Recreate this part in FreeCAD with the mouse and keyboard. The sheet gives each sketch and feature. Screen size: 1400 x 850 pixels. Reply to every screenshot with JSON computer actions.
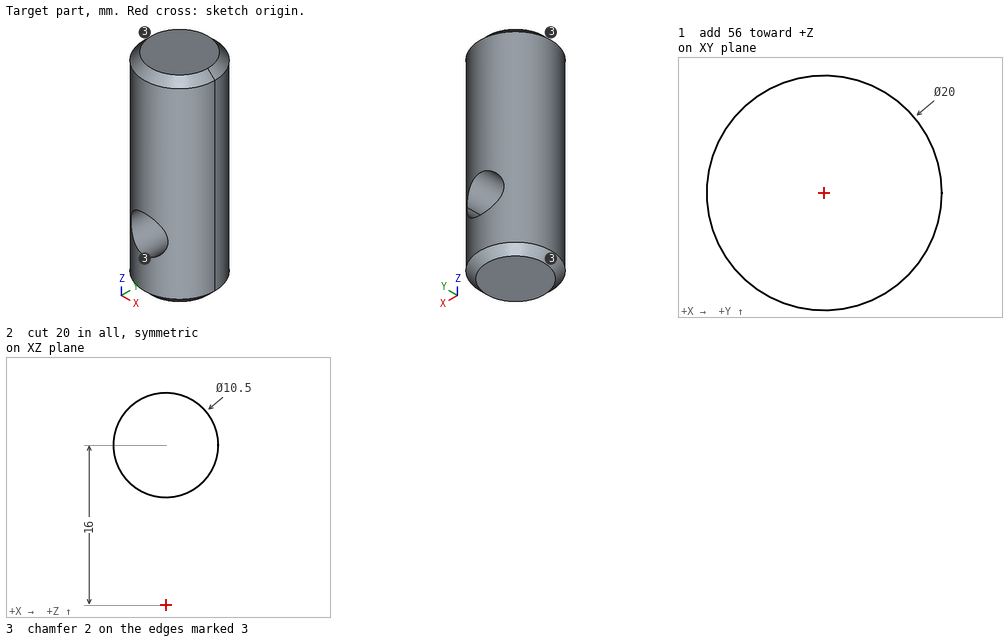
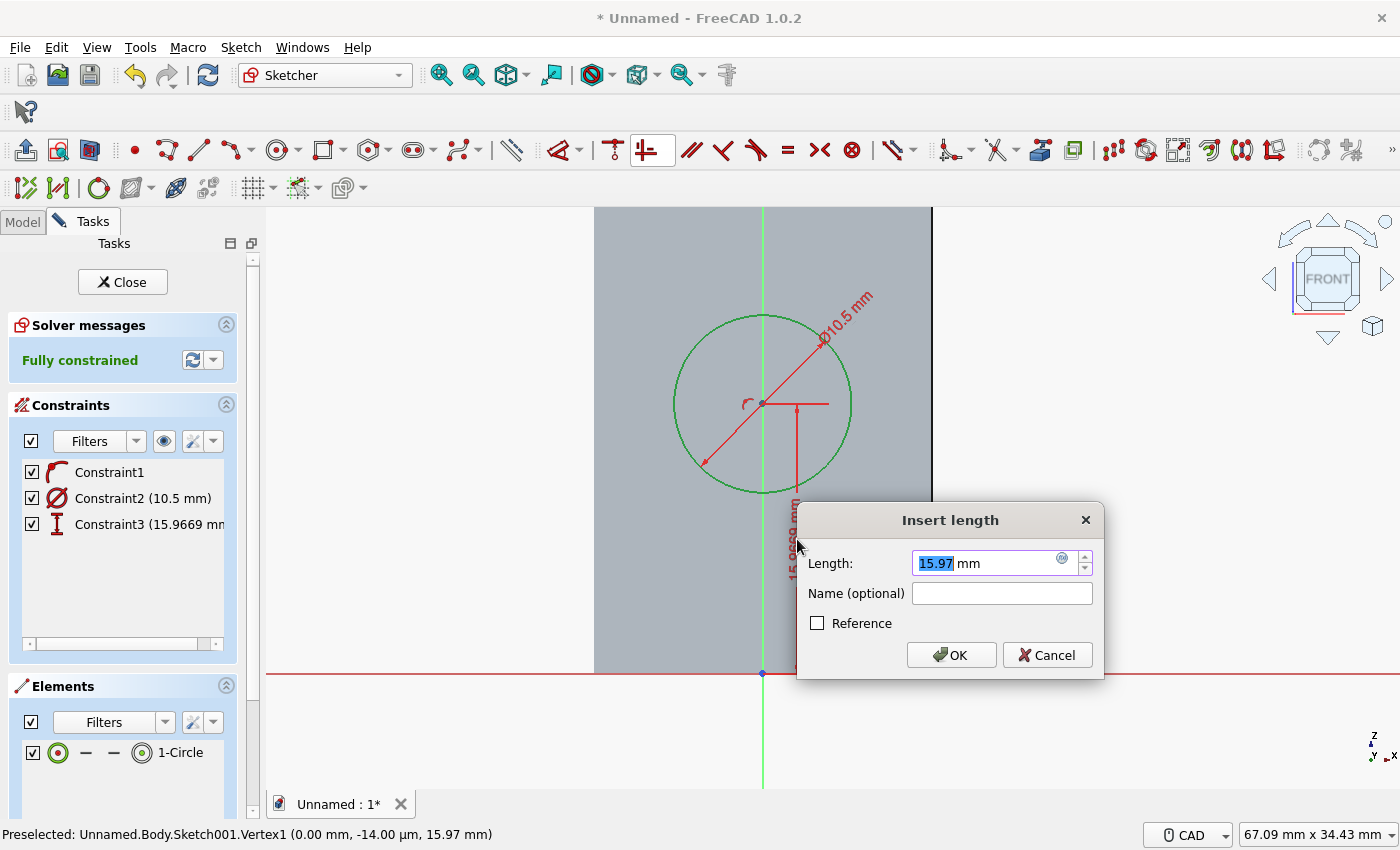
{"action": "type", "text": "16"}
{"action": "key", "text": "Return"}
{"action": "key", "text": "Escape"}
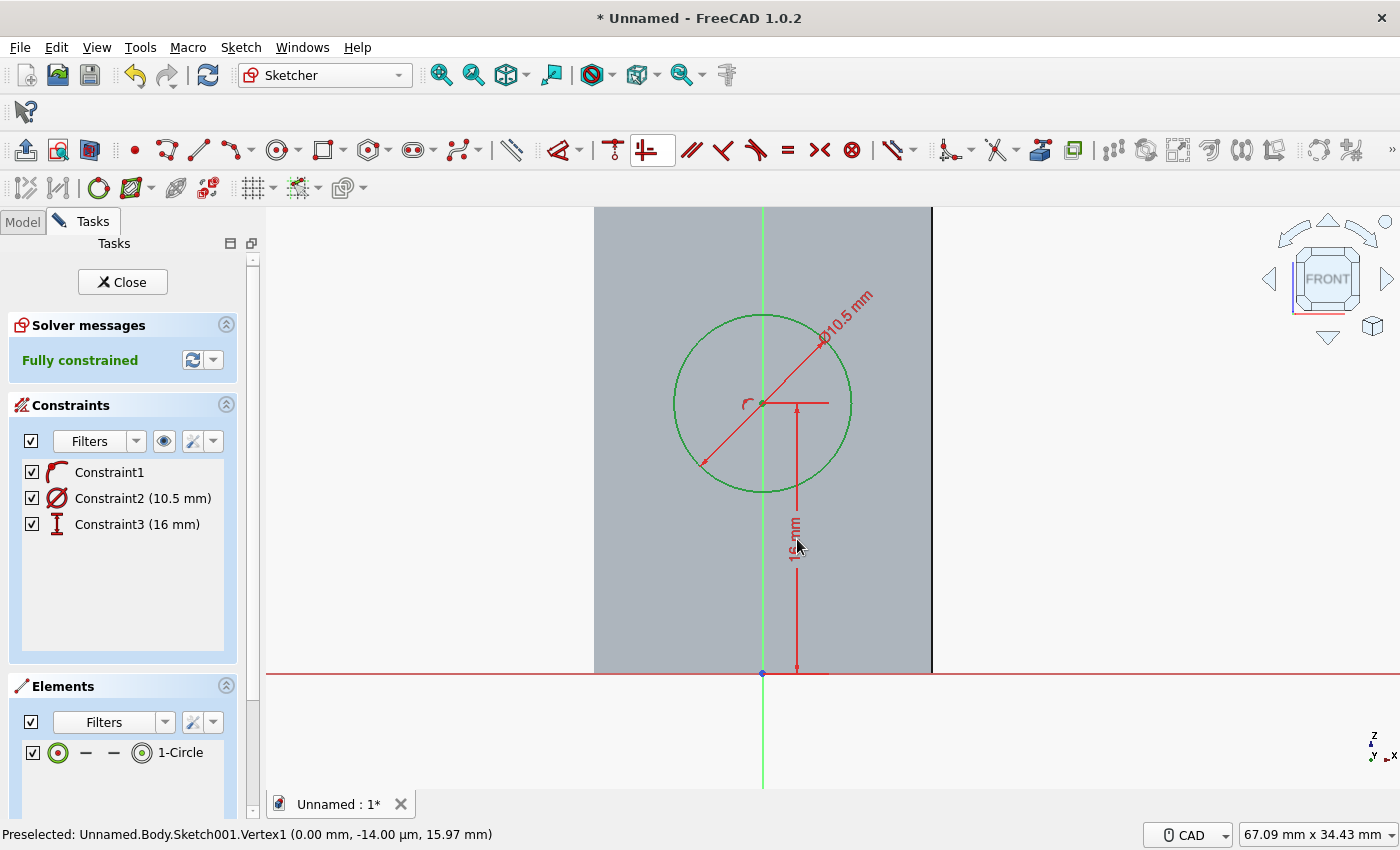
{"action": "left_click", "coordinate": [123, 282]}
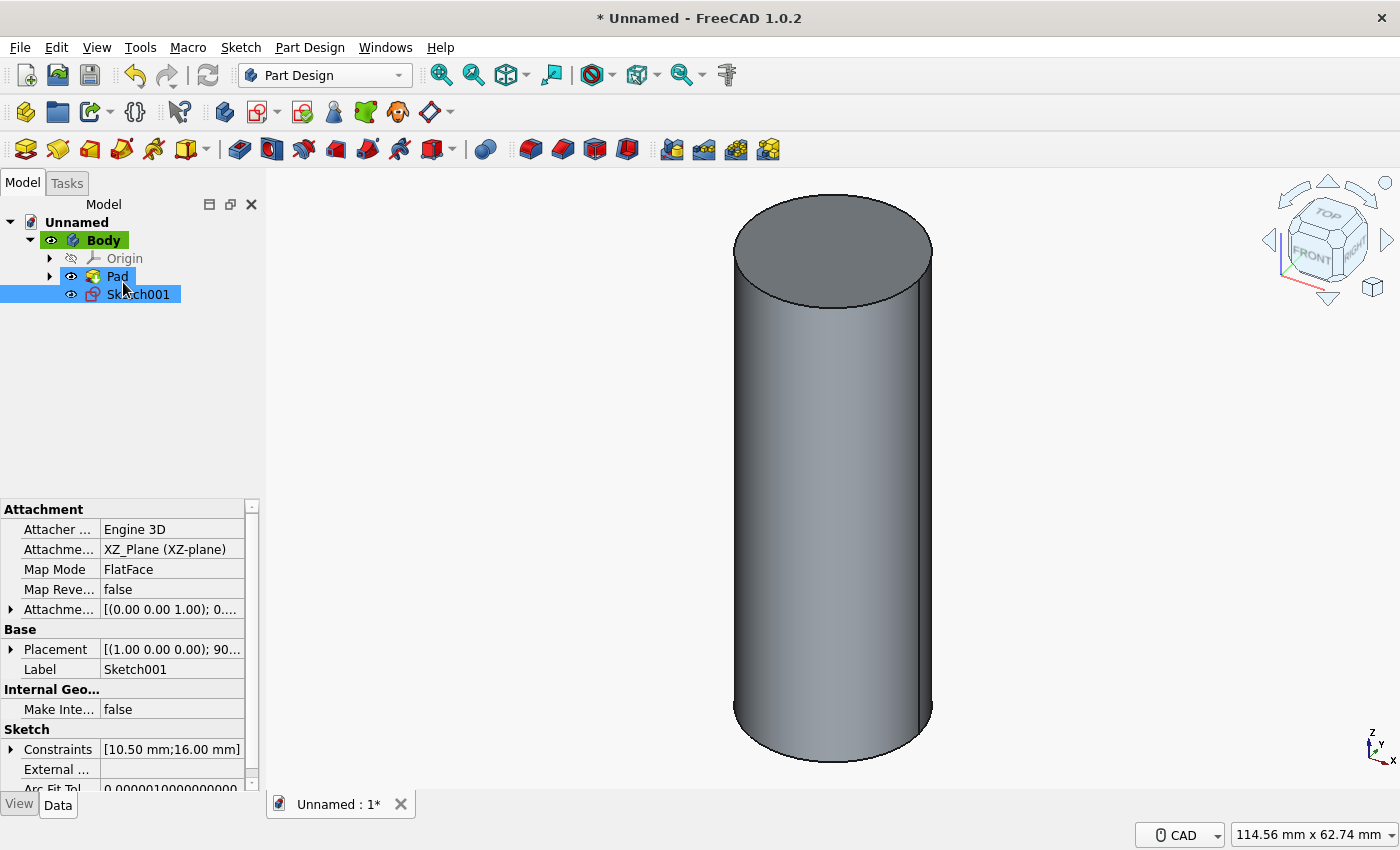
{"action": "left_click", "coordinate": [240, 150]}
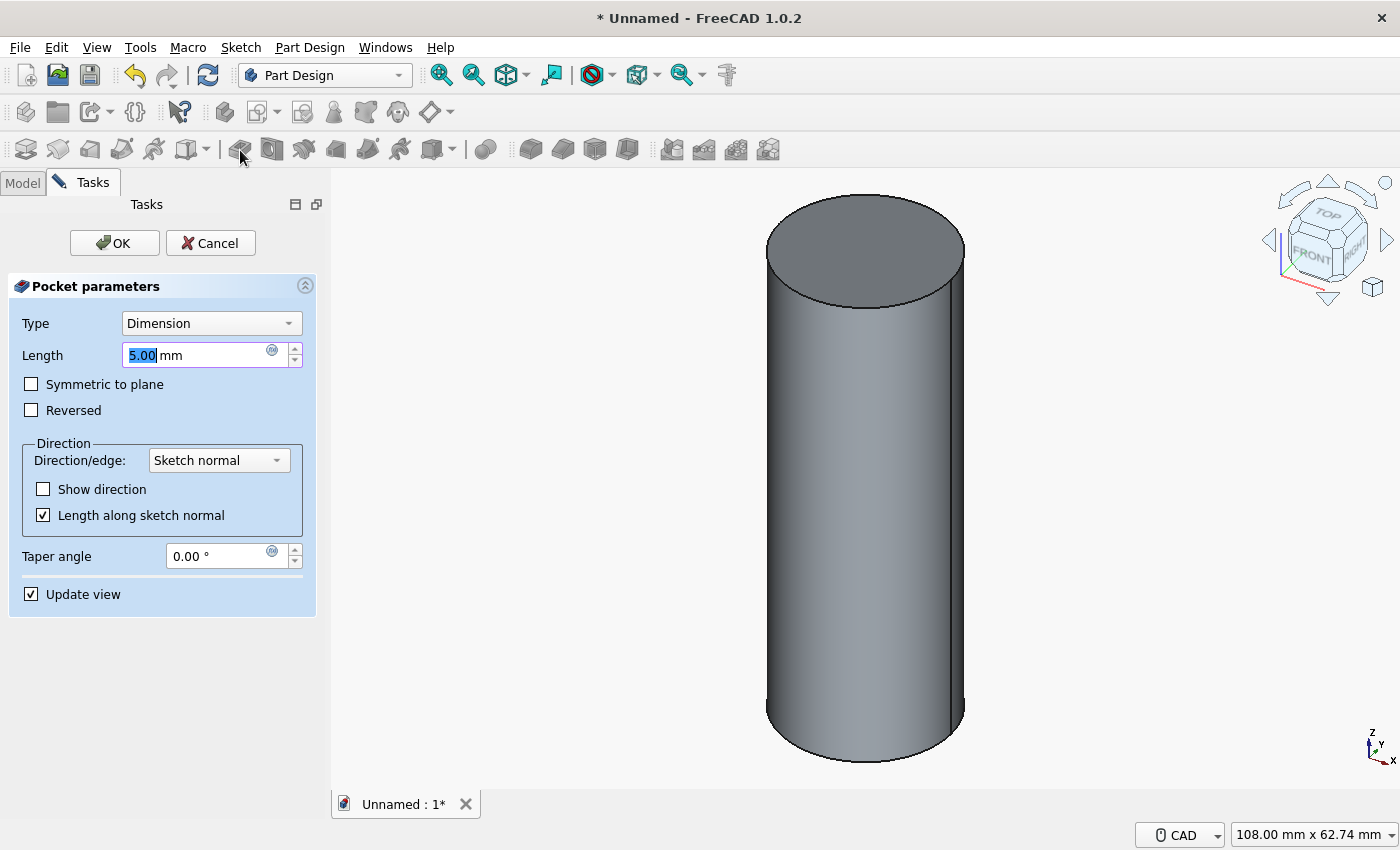
{"action": "type", "text": "20"}
{"action": "key", "text": "Tab"}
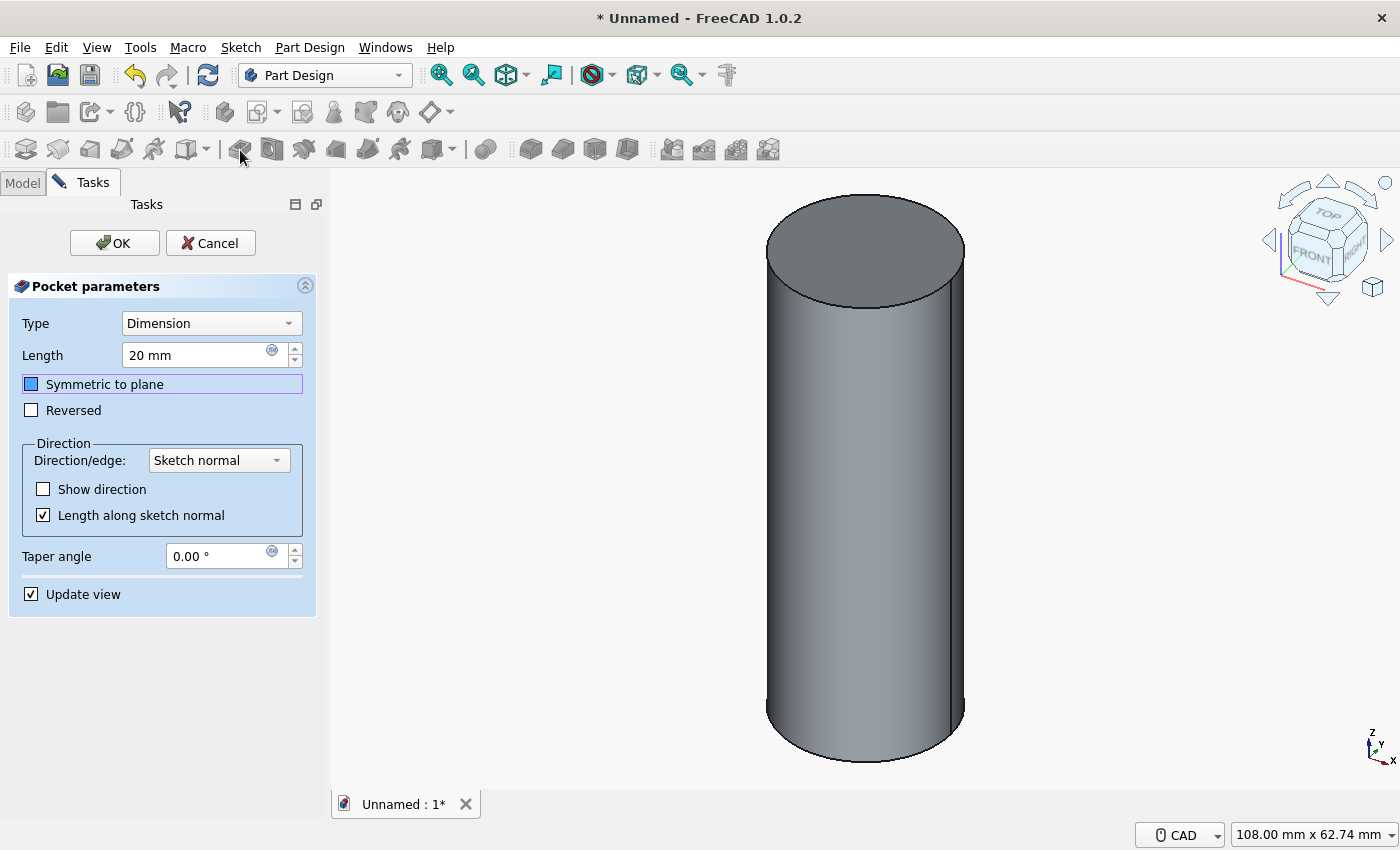
{"action": "left_click", "coordinate": [30, 384]}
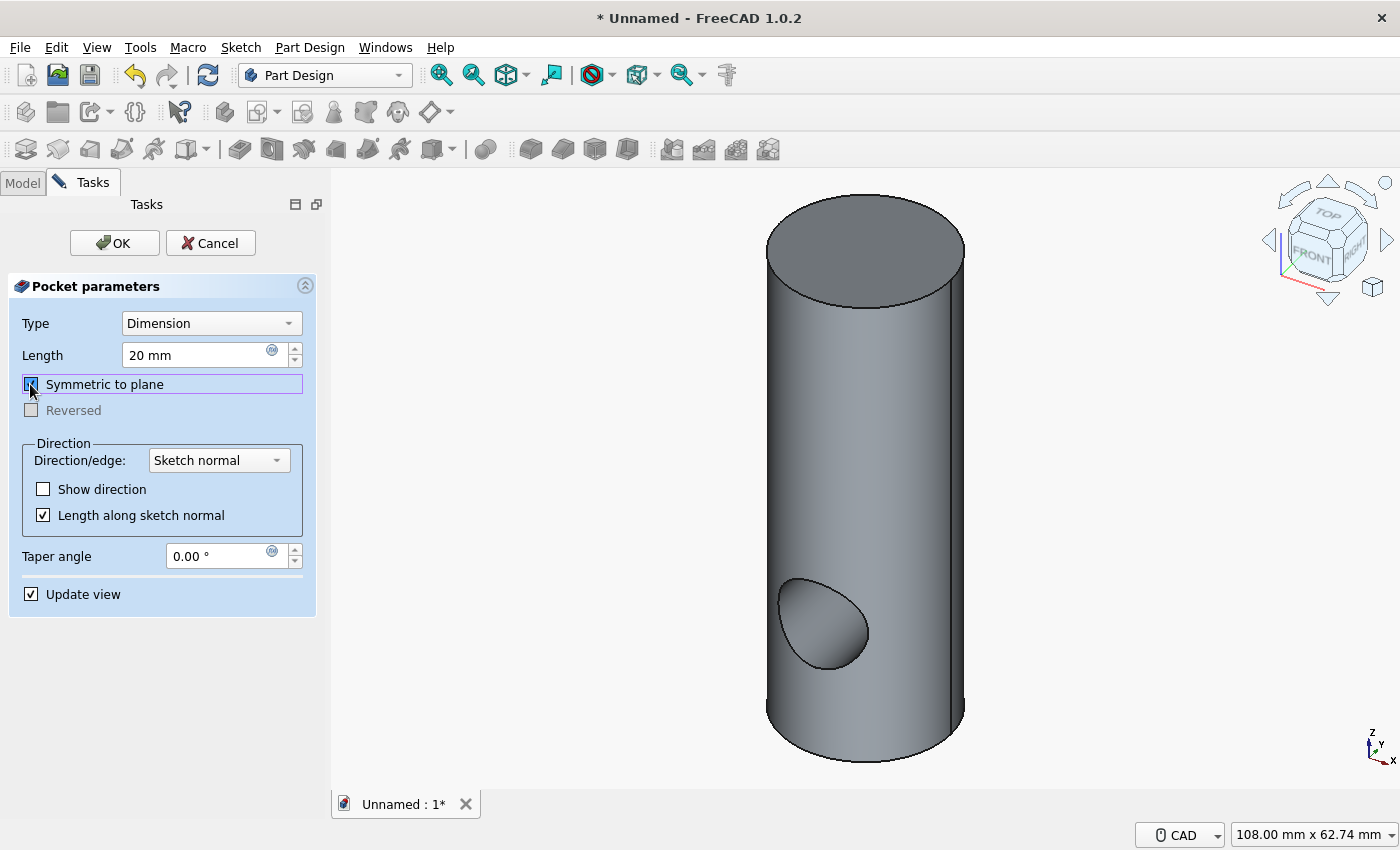
{"action": "left_click", "coordinate": [115, 243]}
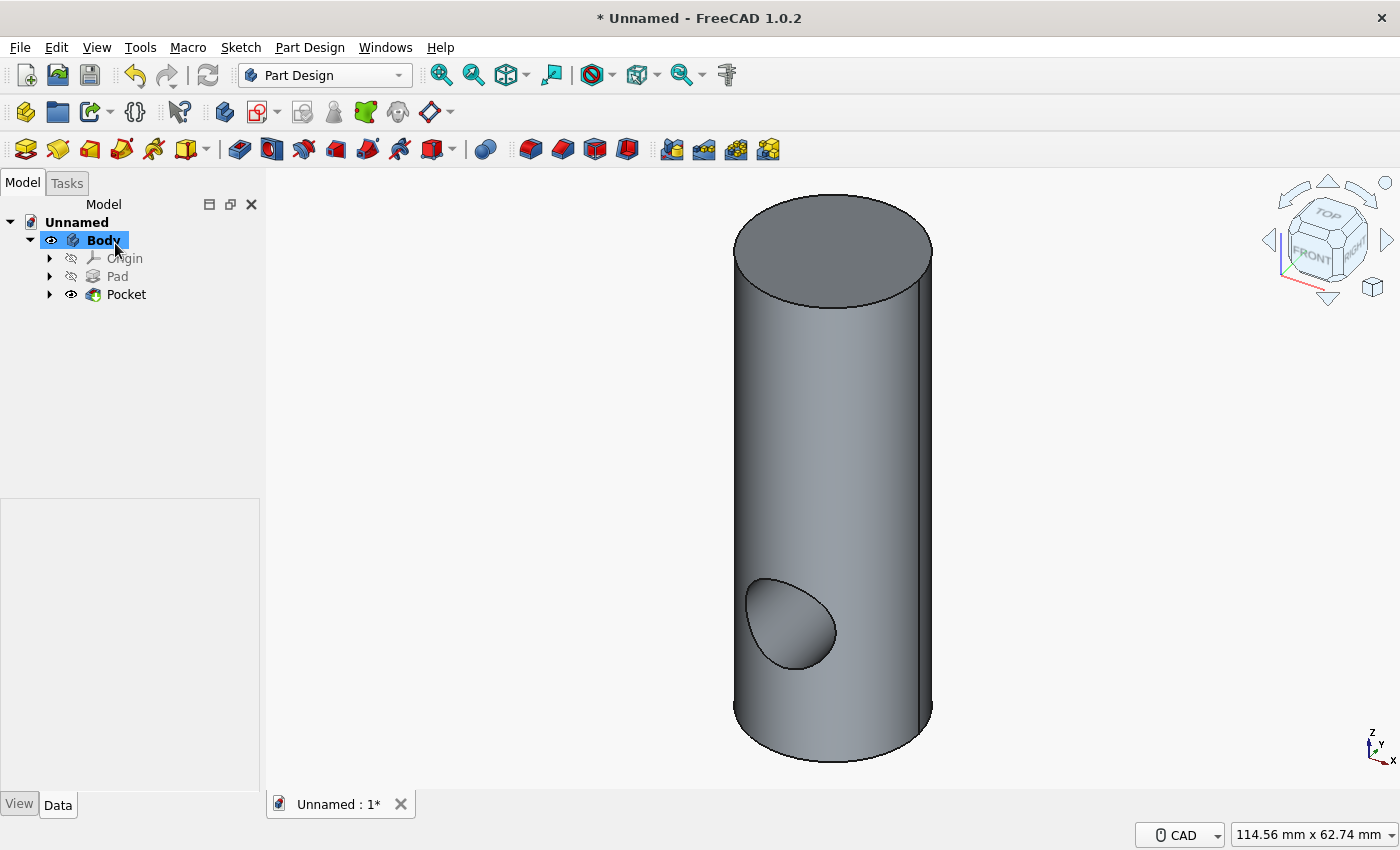
{"action": "left_click", "coordinate": [862, 759]}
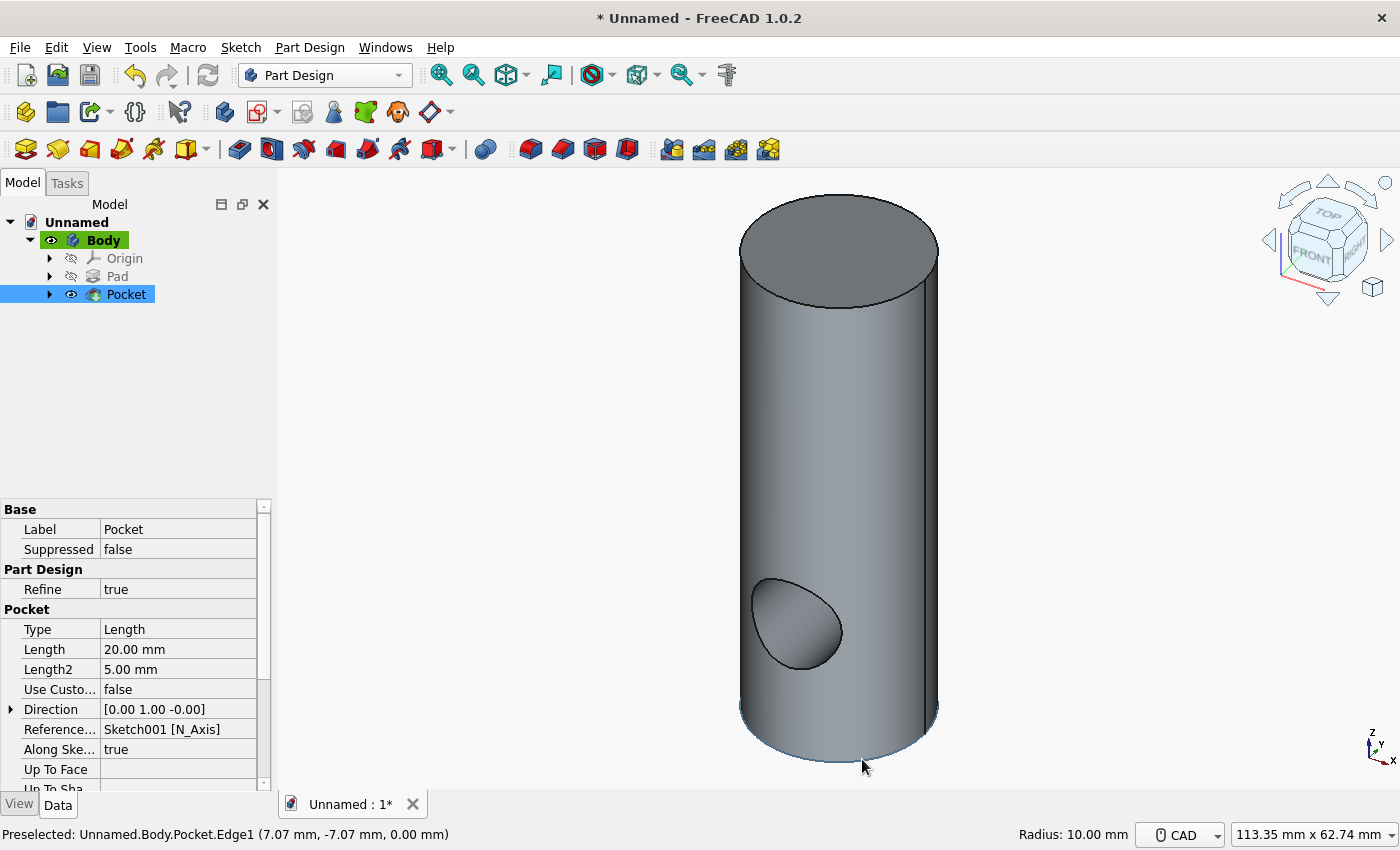
{"action": "left_click", "coordinate": [741, 256], "text": "ctrl"}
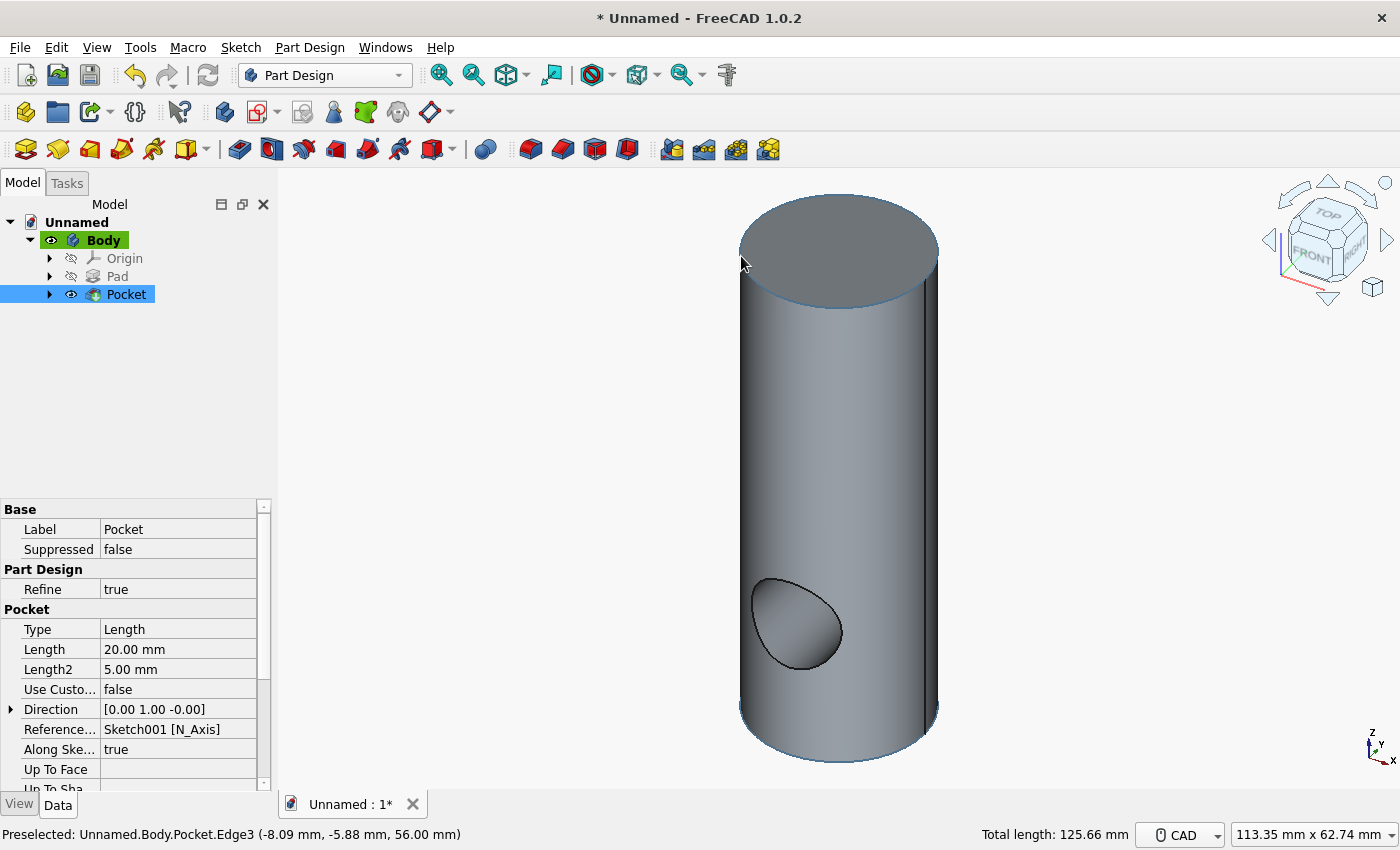
{"action": "left_click", "coordinate": [564, 150]}